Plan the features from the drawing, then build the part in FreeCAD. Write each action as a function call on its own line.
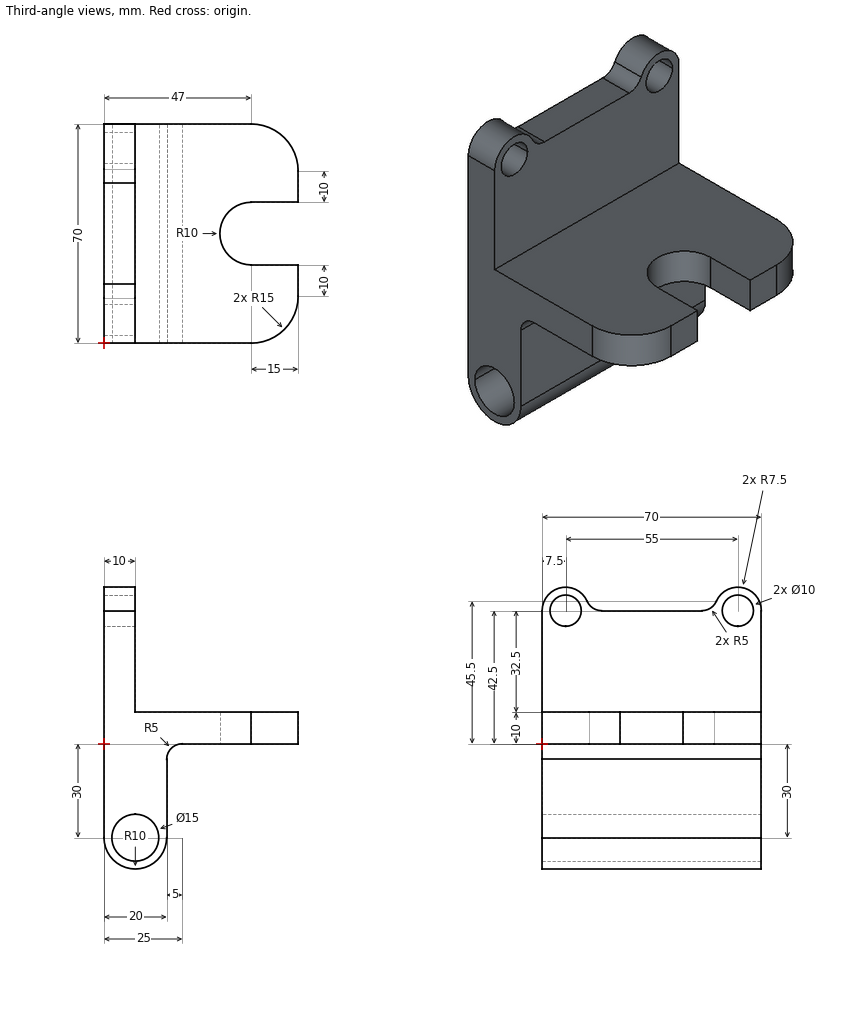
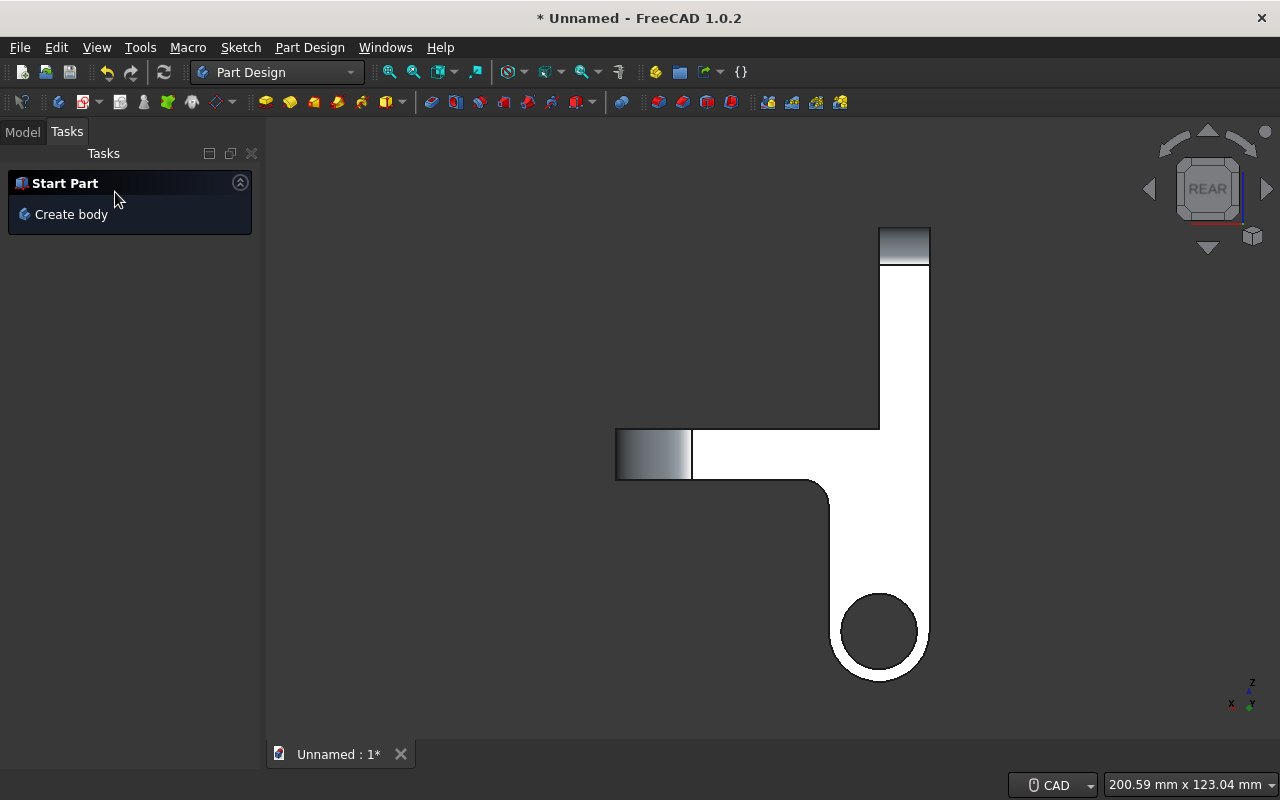
key(0)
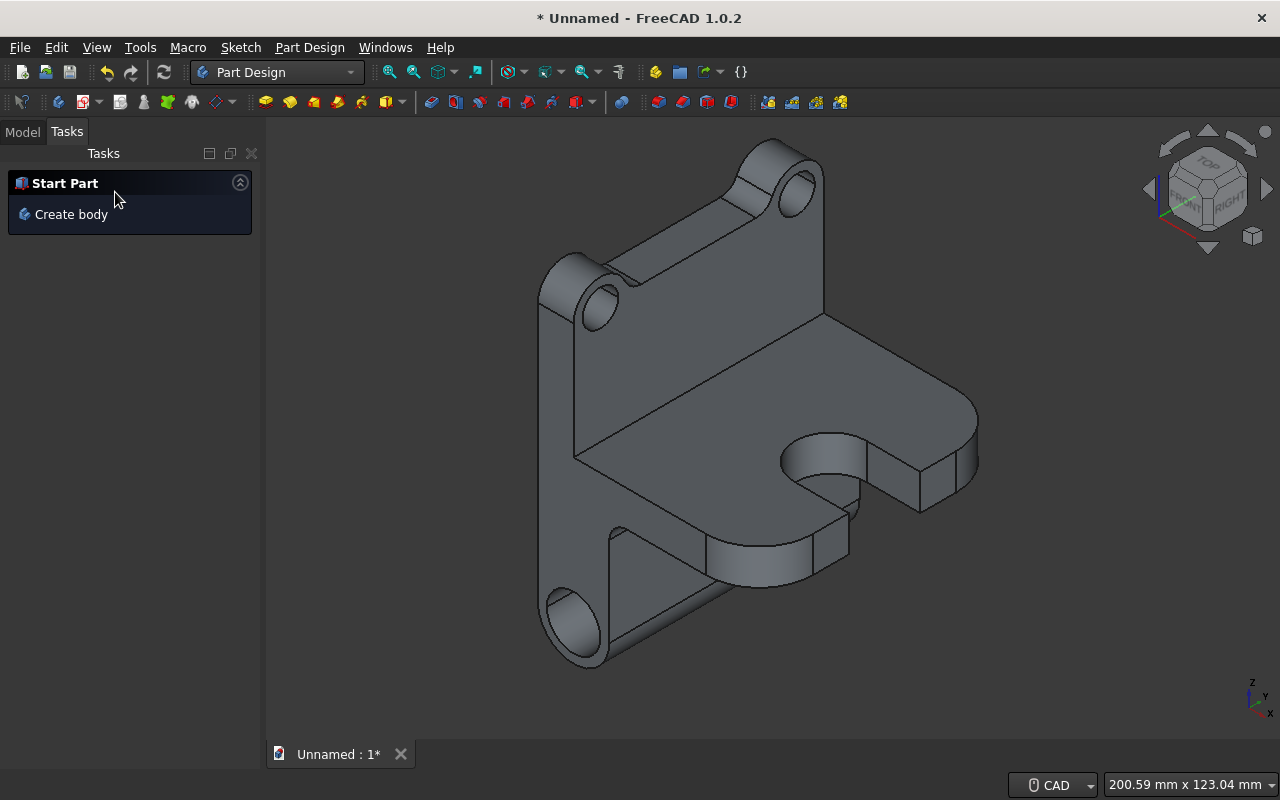
click(390, 72)